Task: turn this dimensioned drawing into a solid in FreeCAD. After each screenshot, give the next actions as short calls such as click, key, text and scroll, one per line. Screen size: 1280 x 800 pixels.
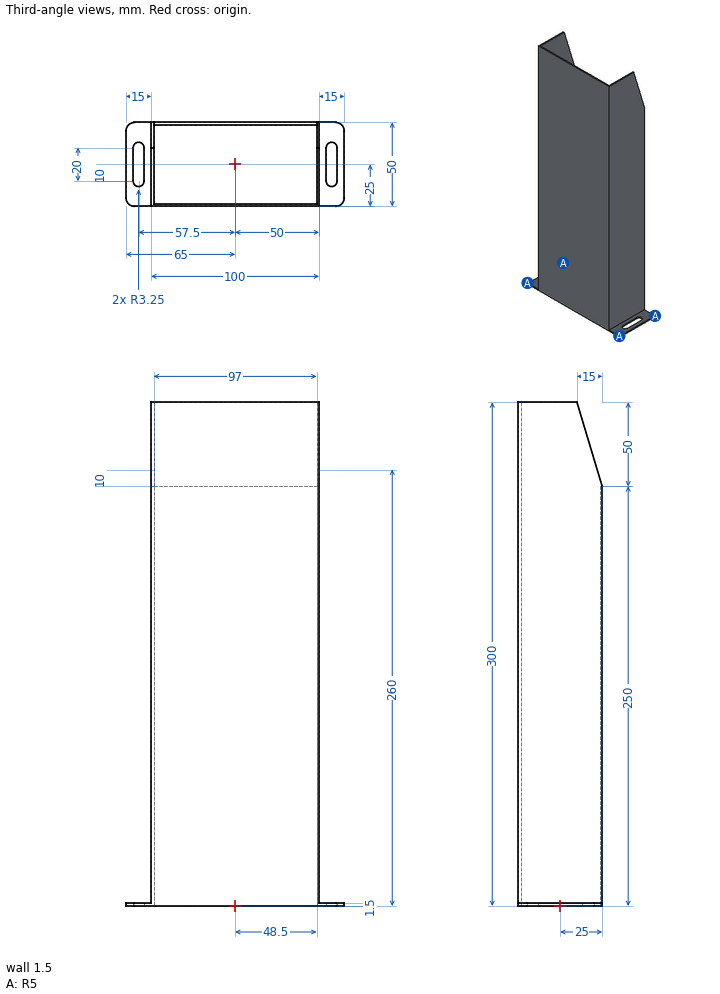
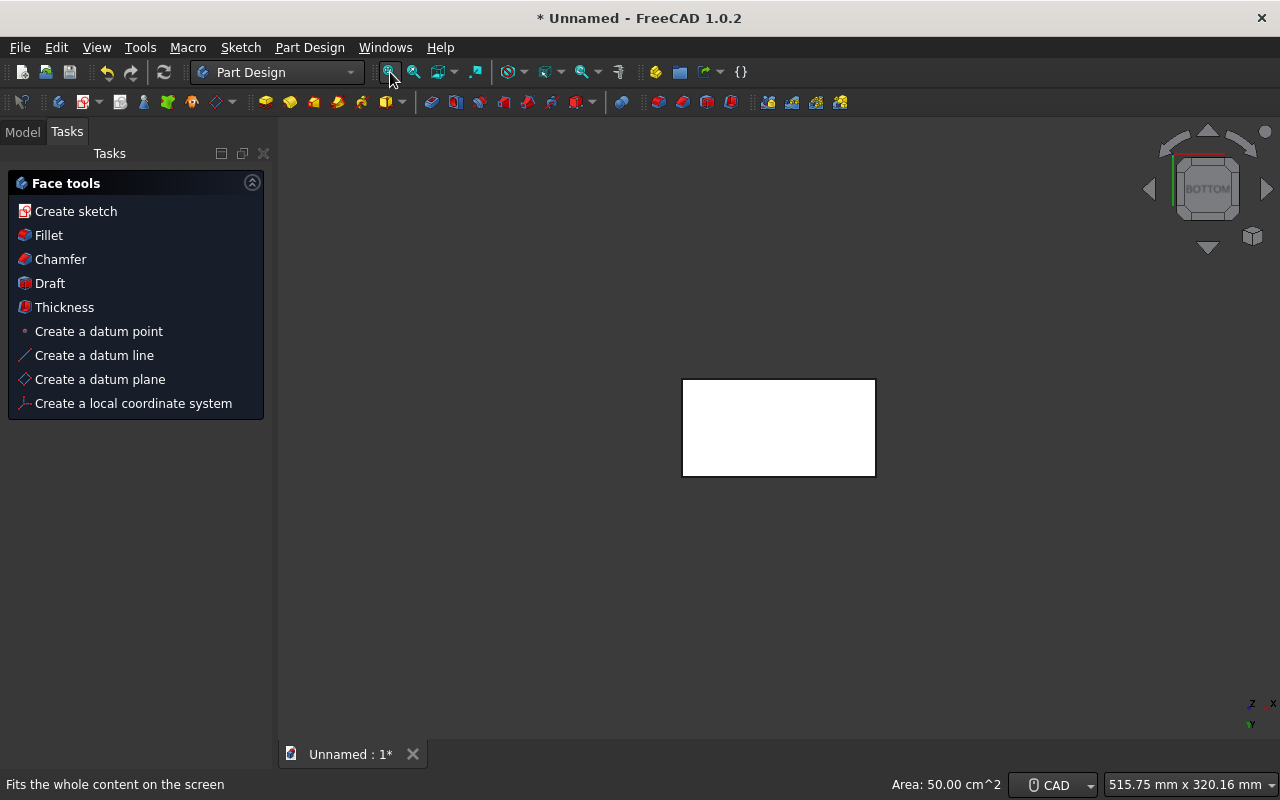
click(390, 72)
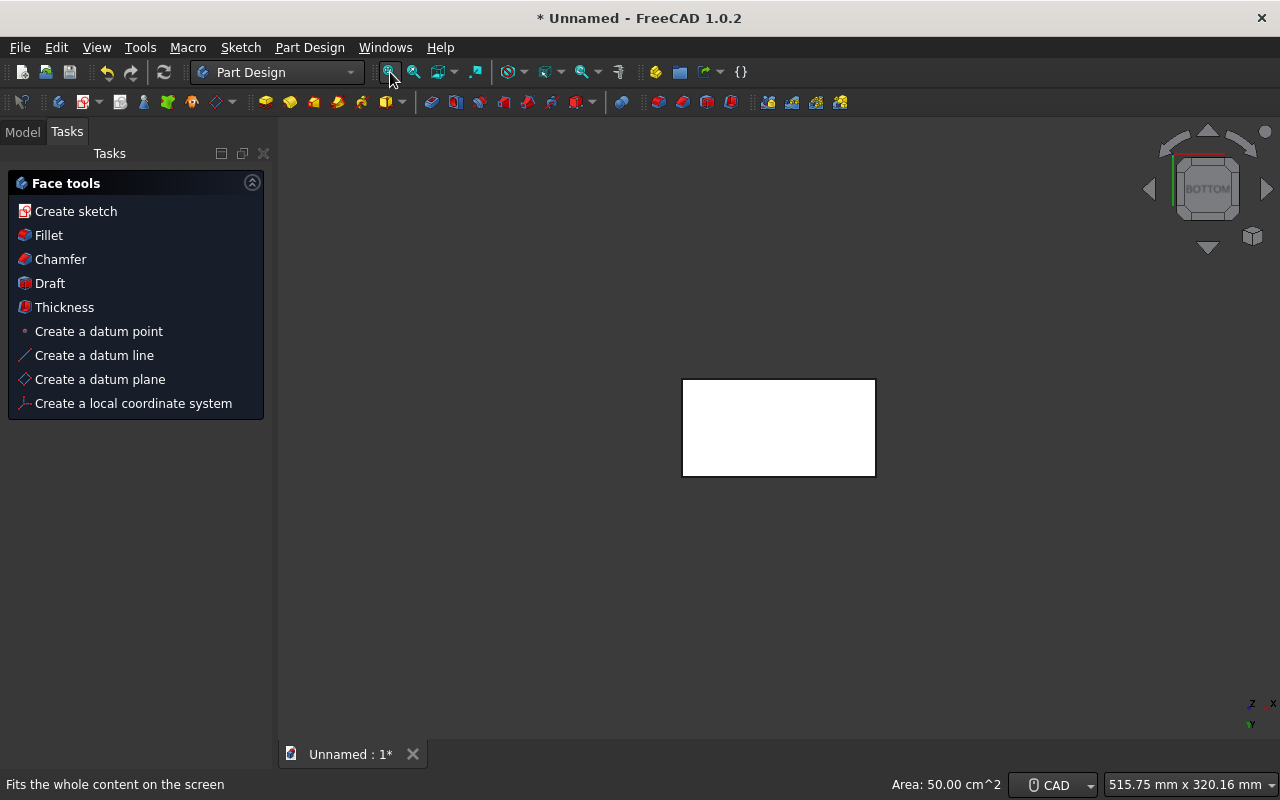
click(807, 427, ctrl)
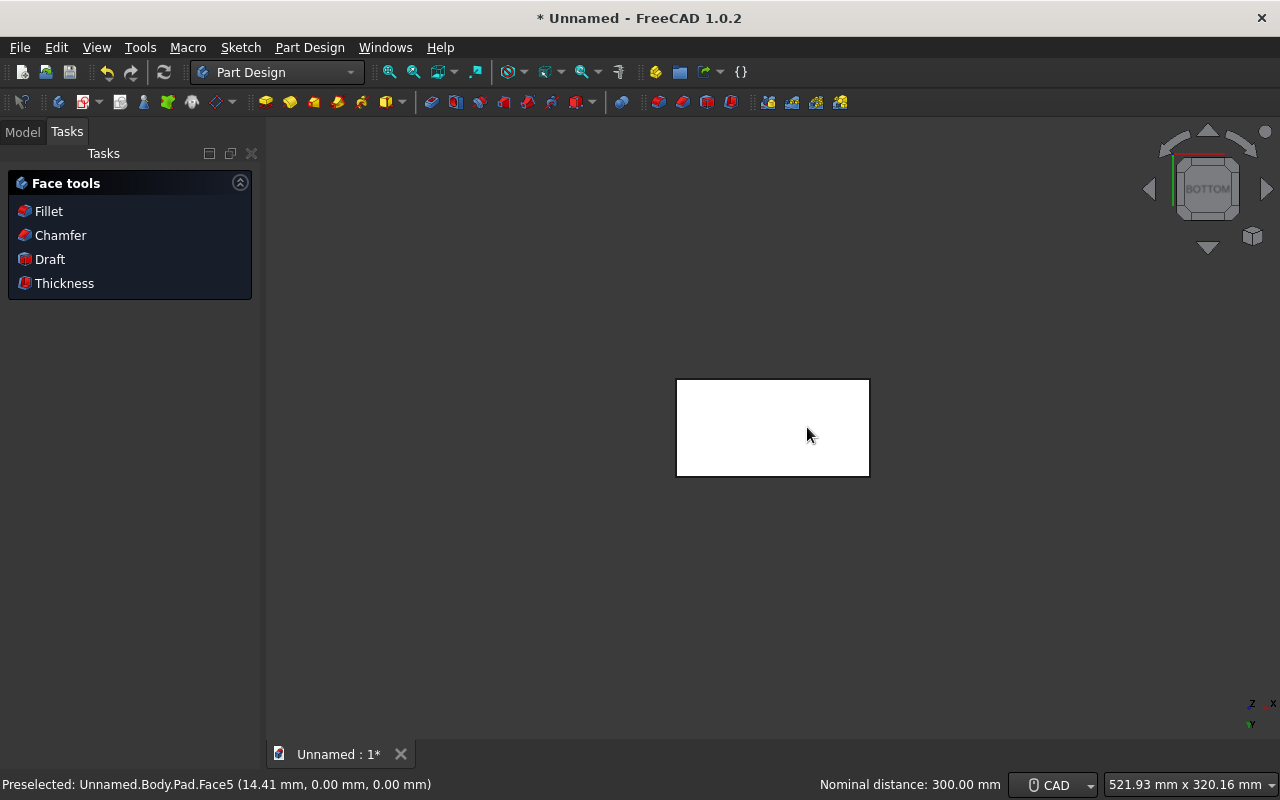
click(732, 102)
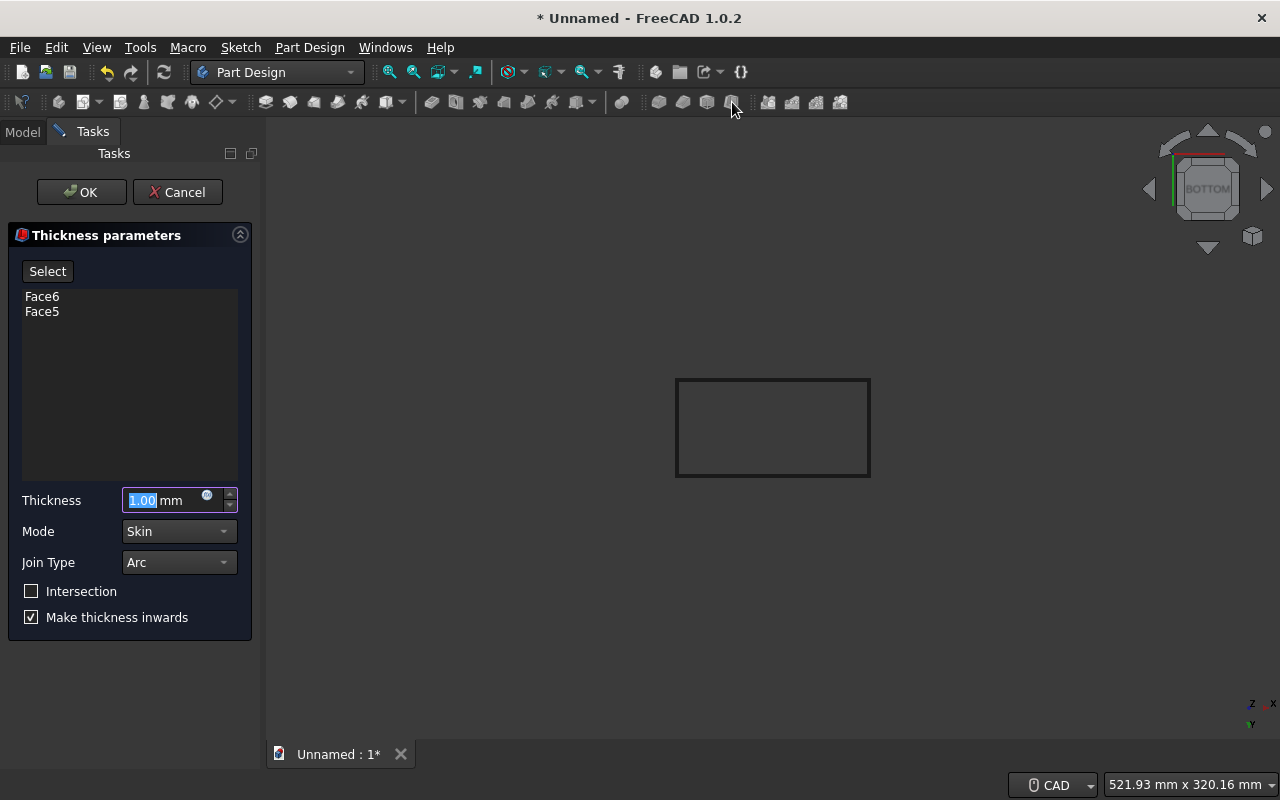
text(1.5)
key(Tab)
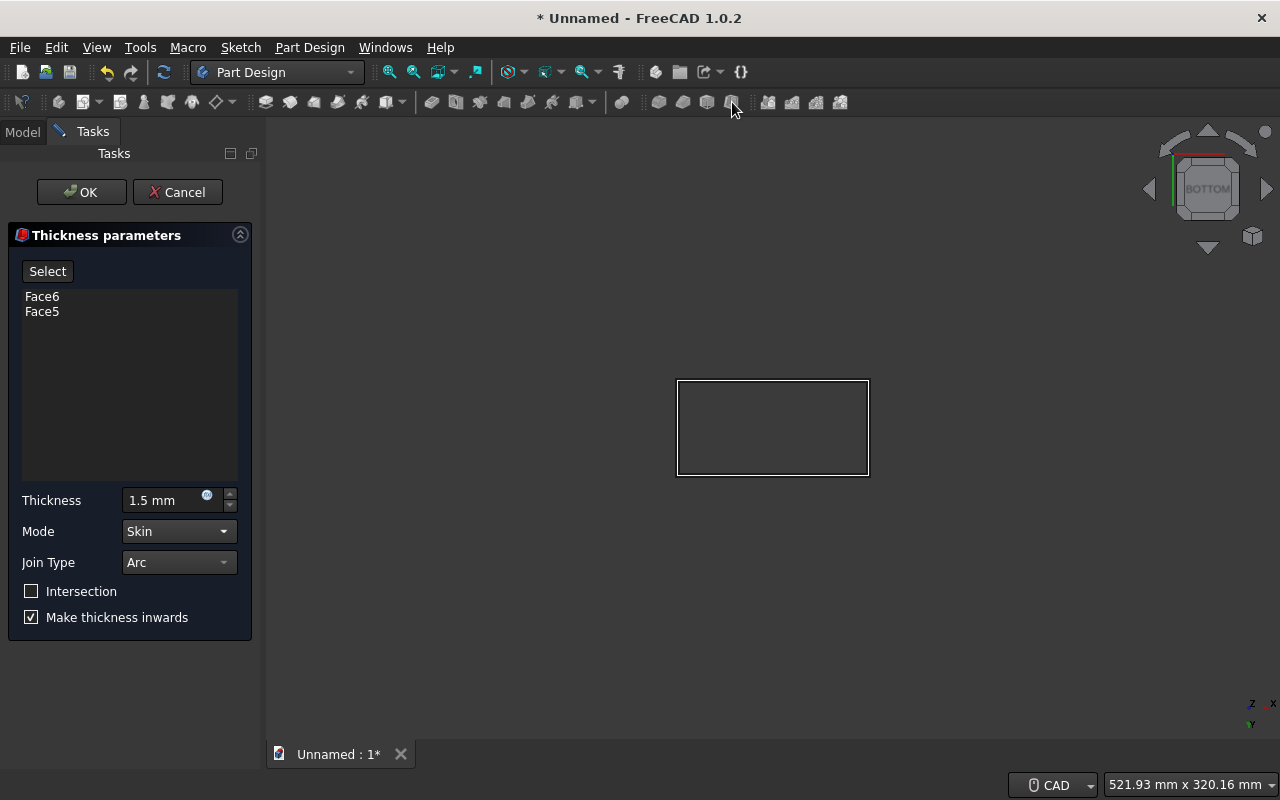
click(180, 562)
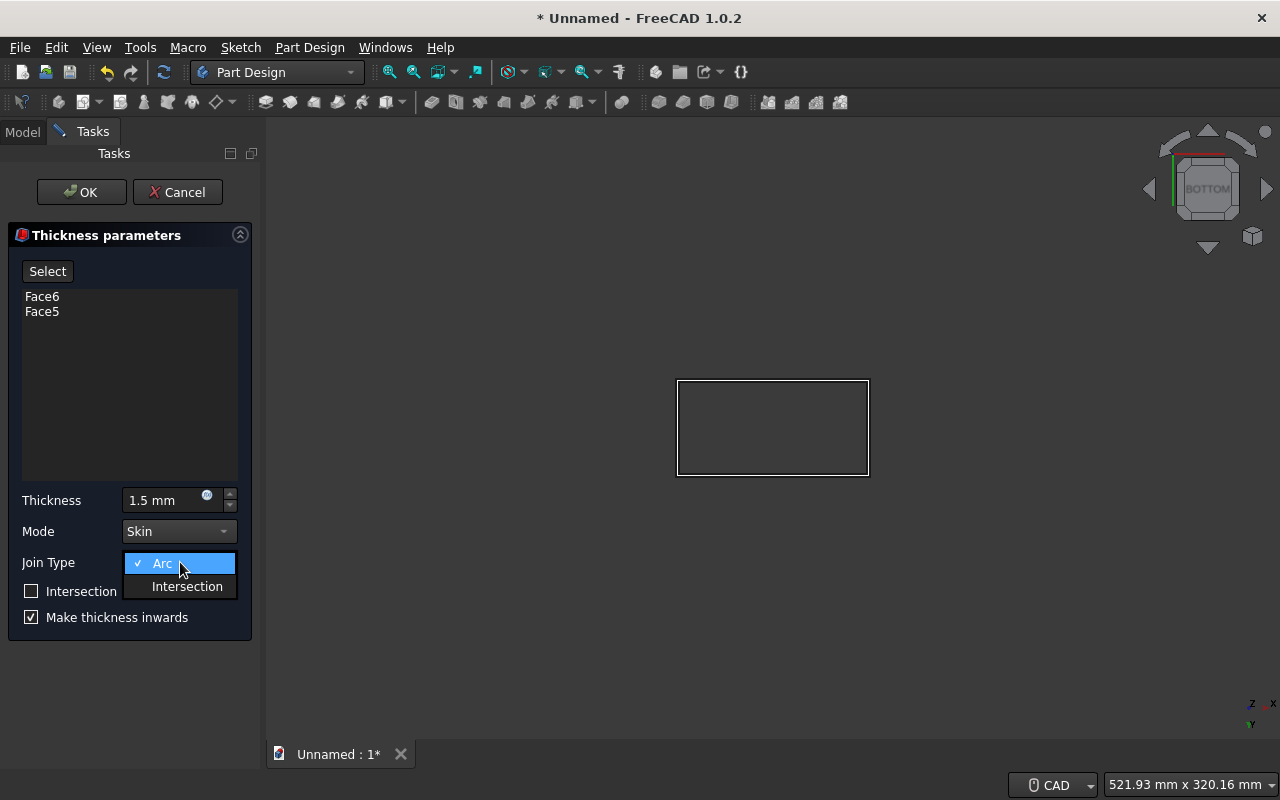
click(179, 586)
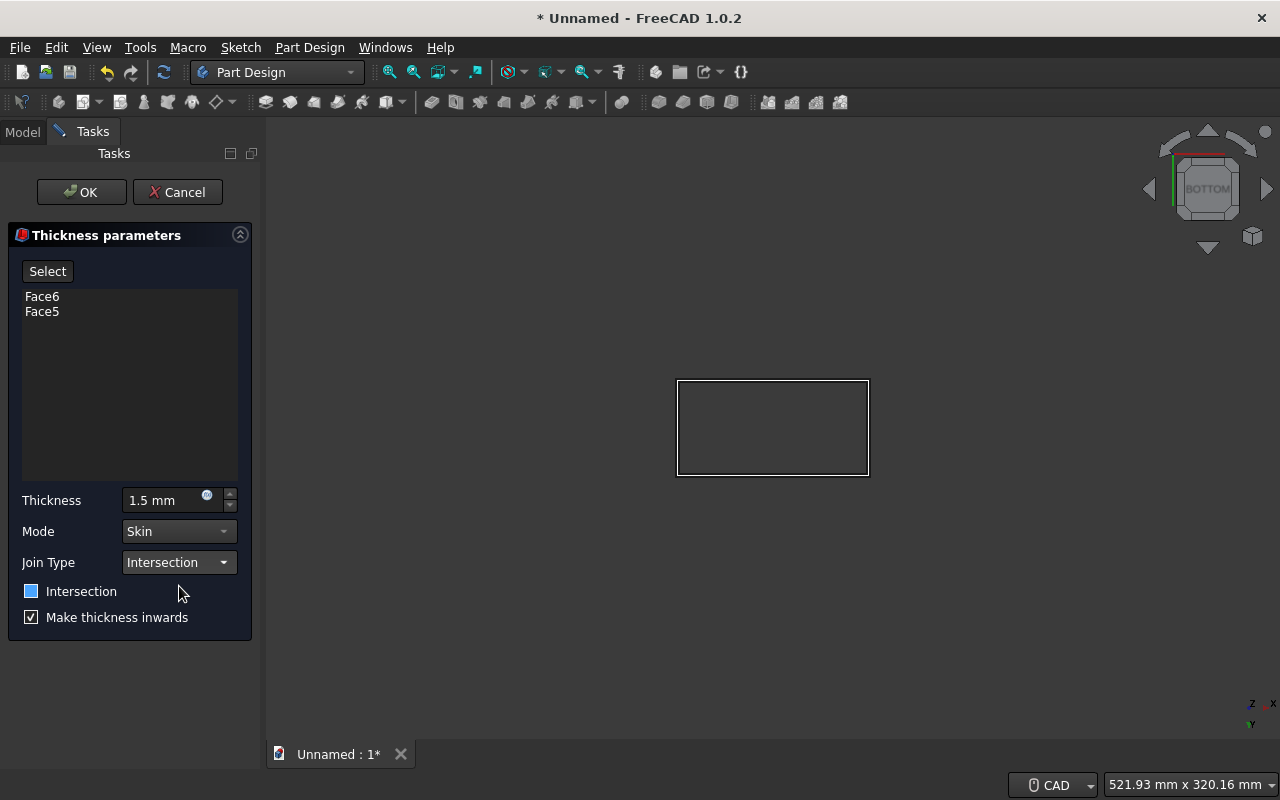
click(82, 192)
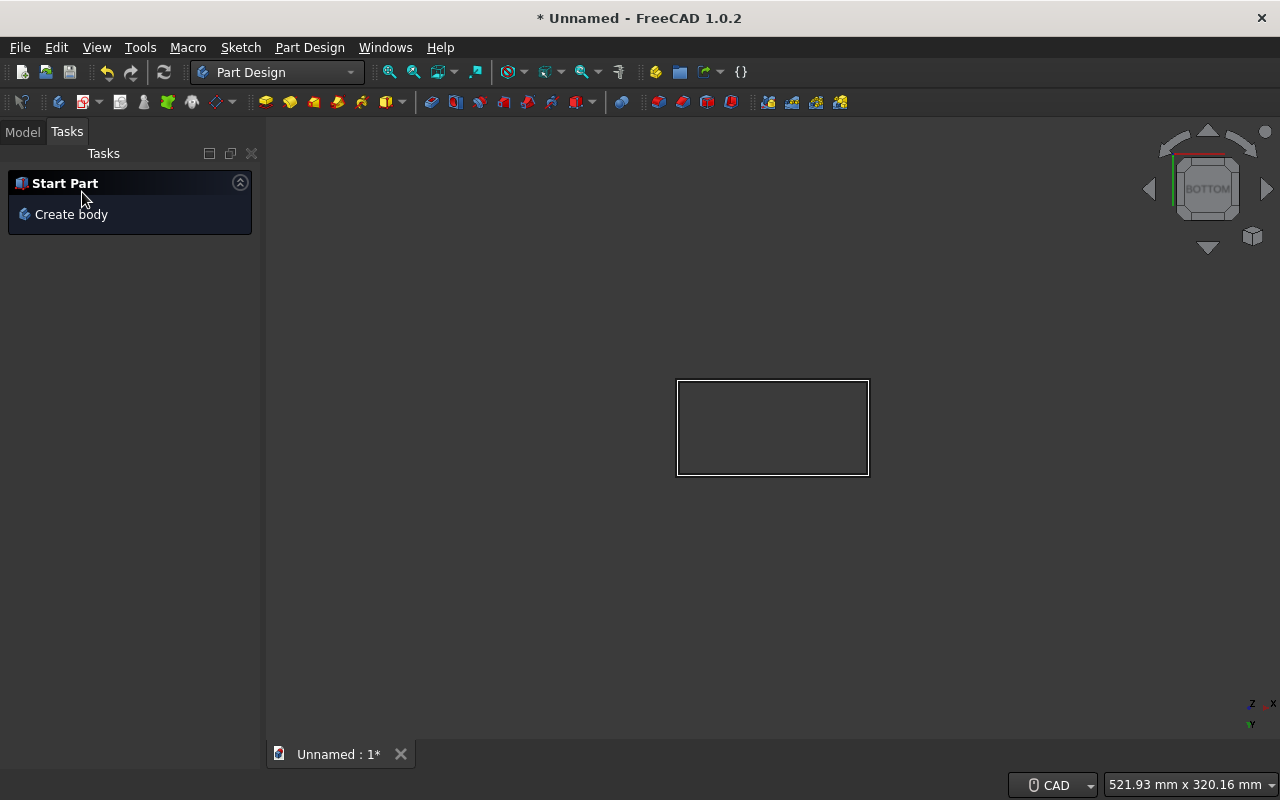
click(390, 72)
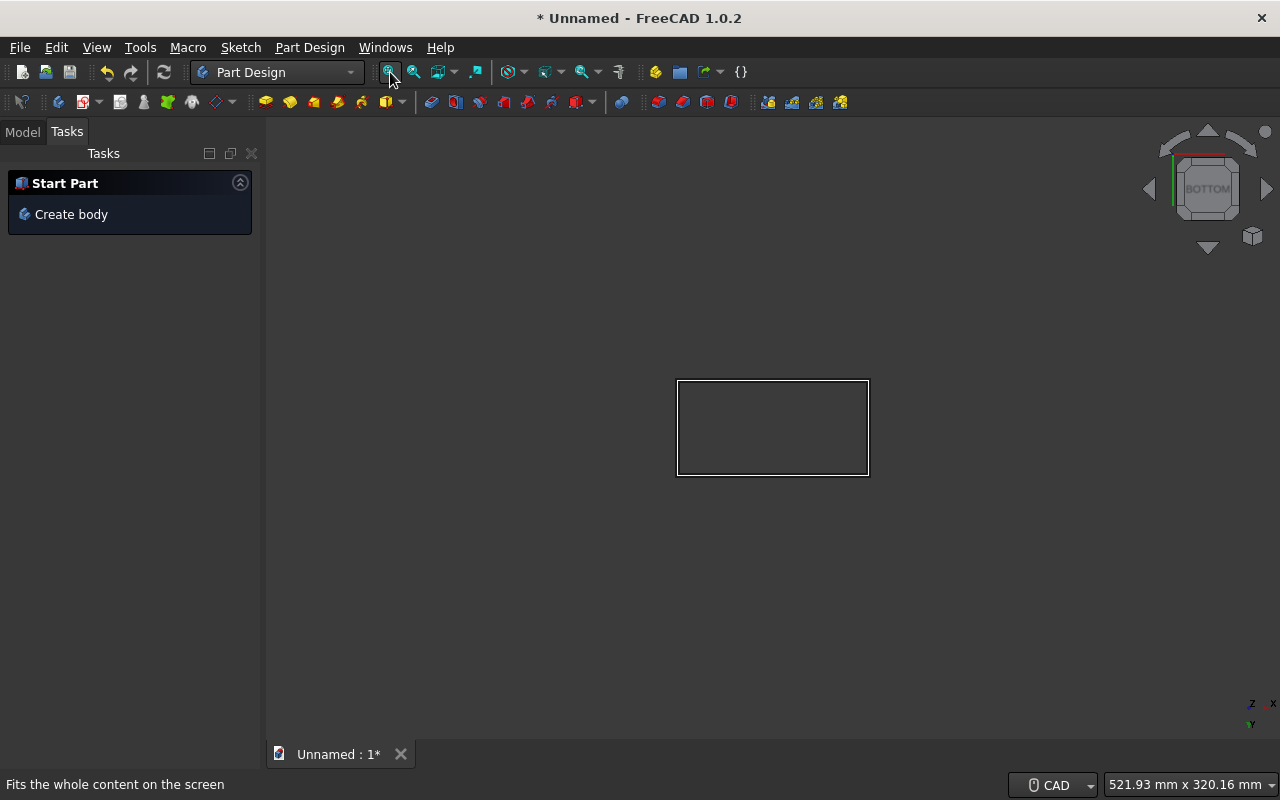
scroll(869, 412, up, 13)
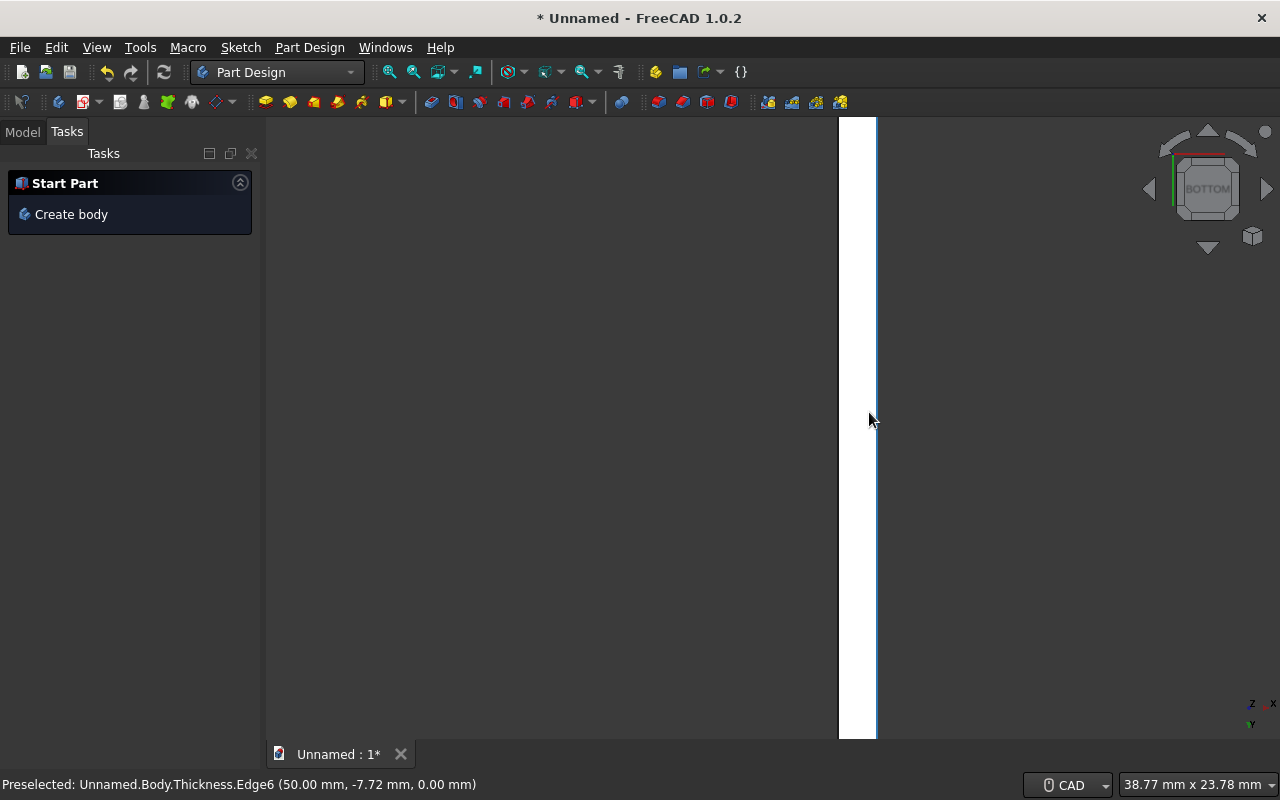
click(864, 416)